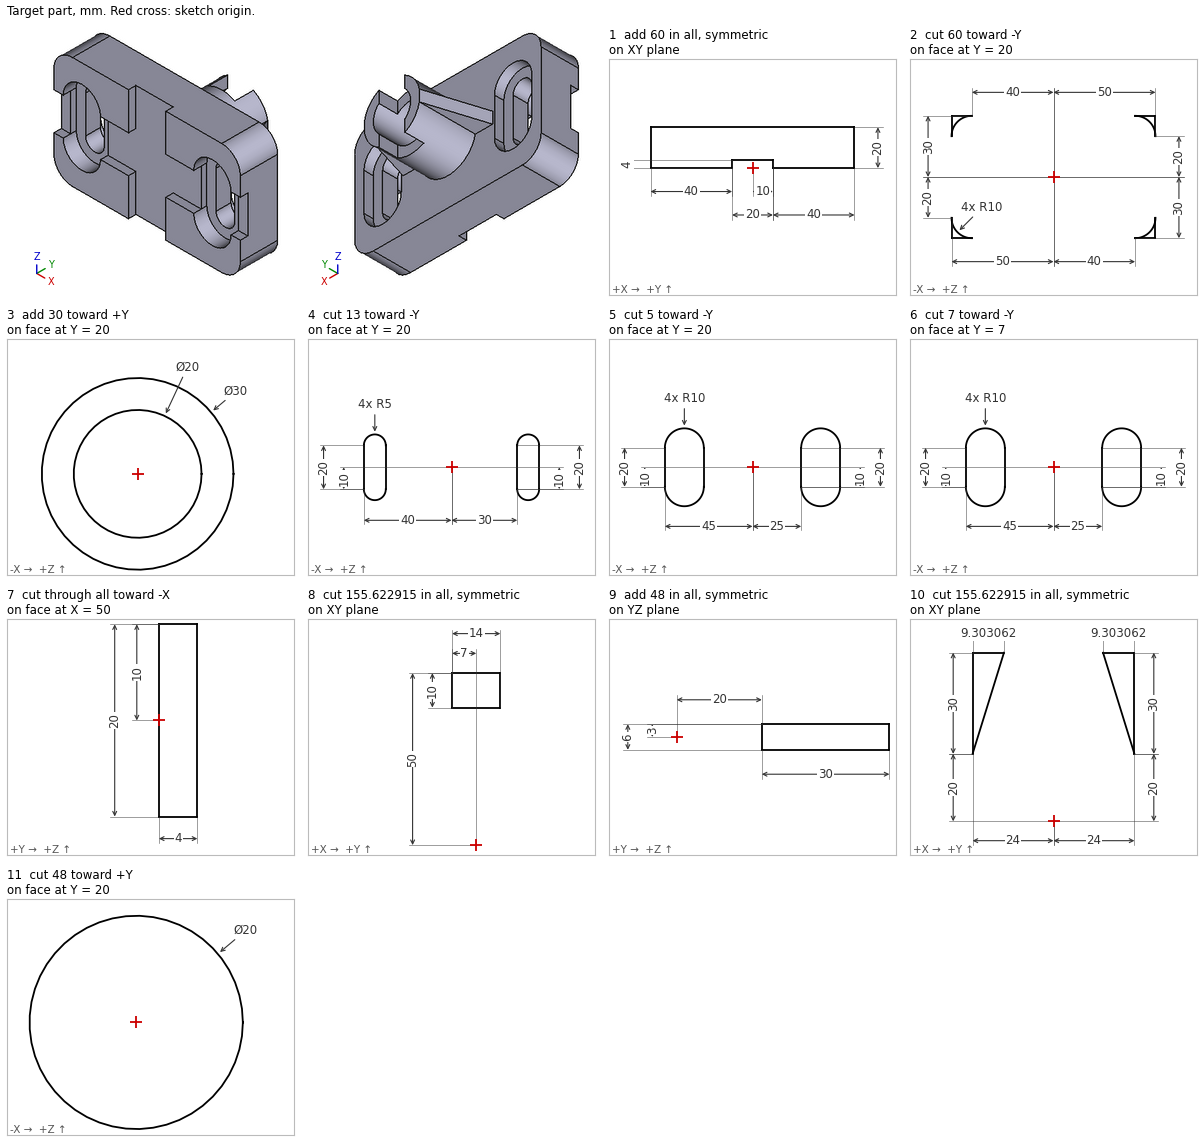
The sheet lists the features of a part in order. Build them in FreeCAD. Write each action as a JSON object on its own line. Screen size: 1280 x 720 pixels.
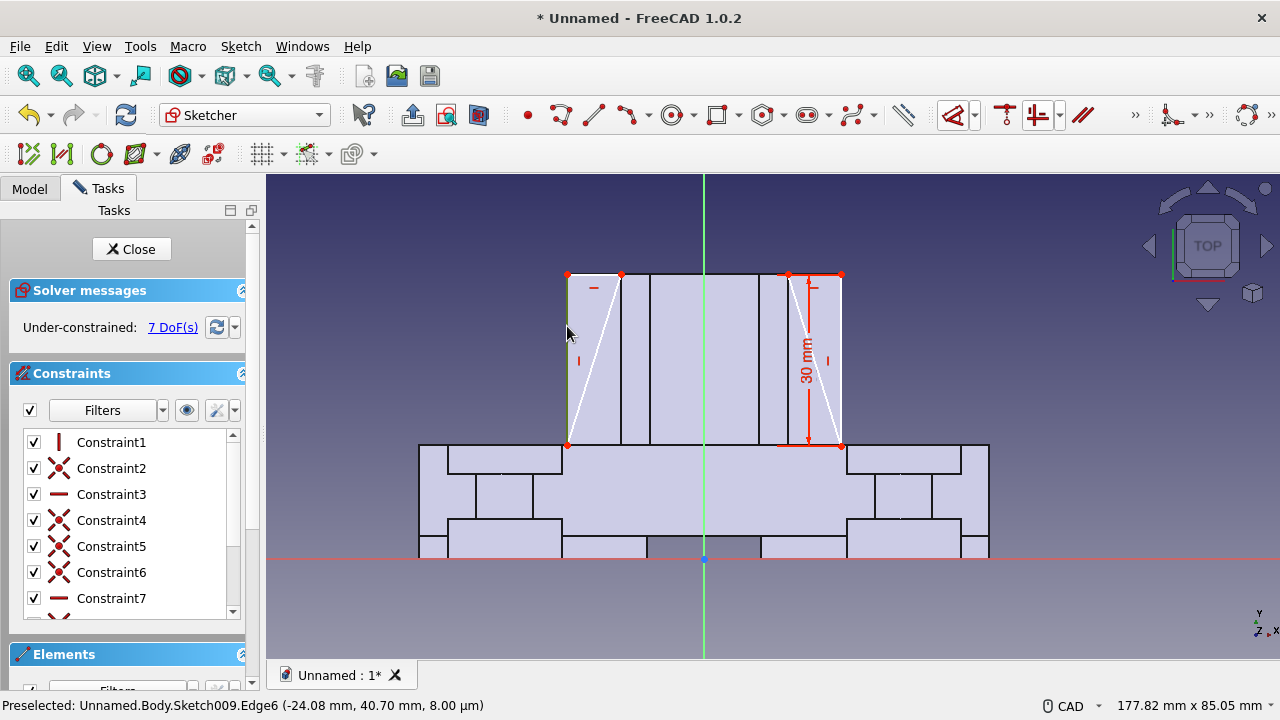
{"action": "left_click", "coordinate": [974, 116]}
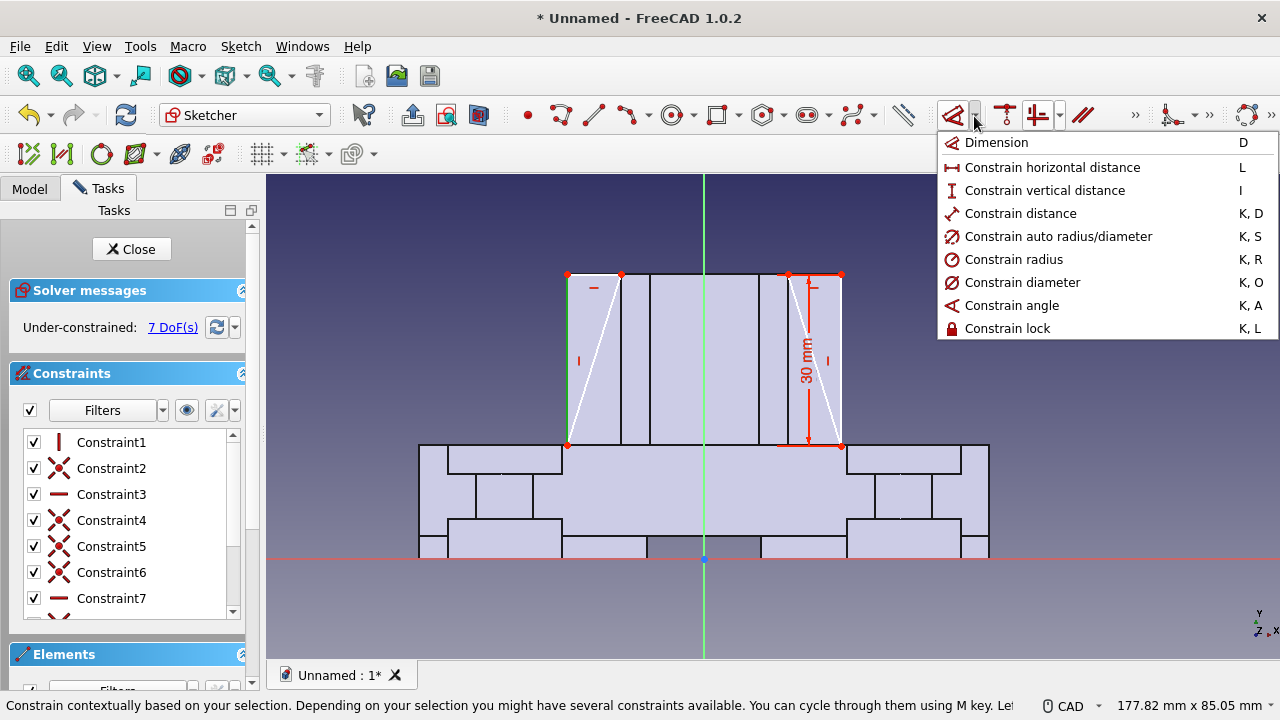
{"action": "left_click", "coordinate": [1108, 190]}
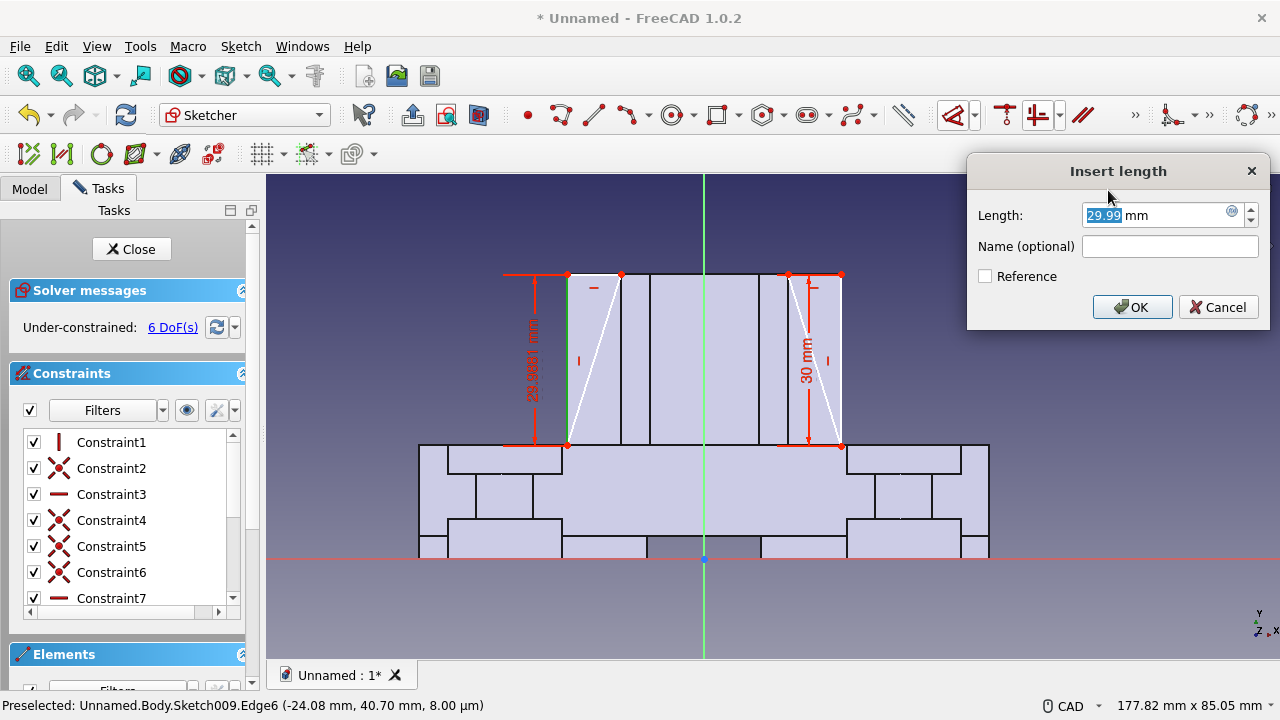
{"action": "type", "text": "30"}
{"action": "key", "text": "Return"}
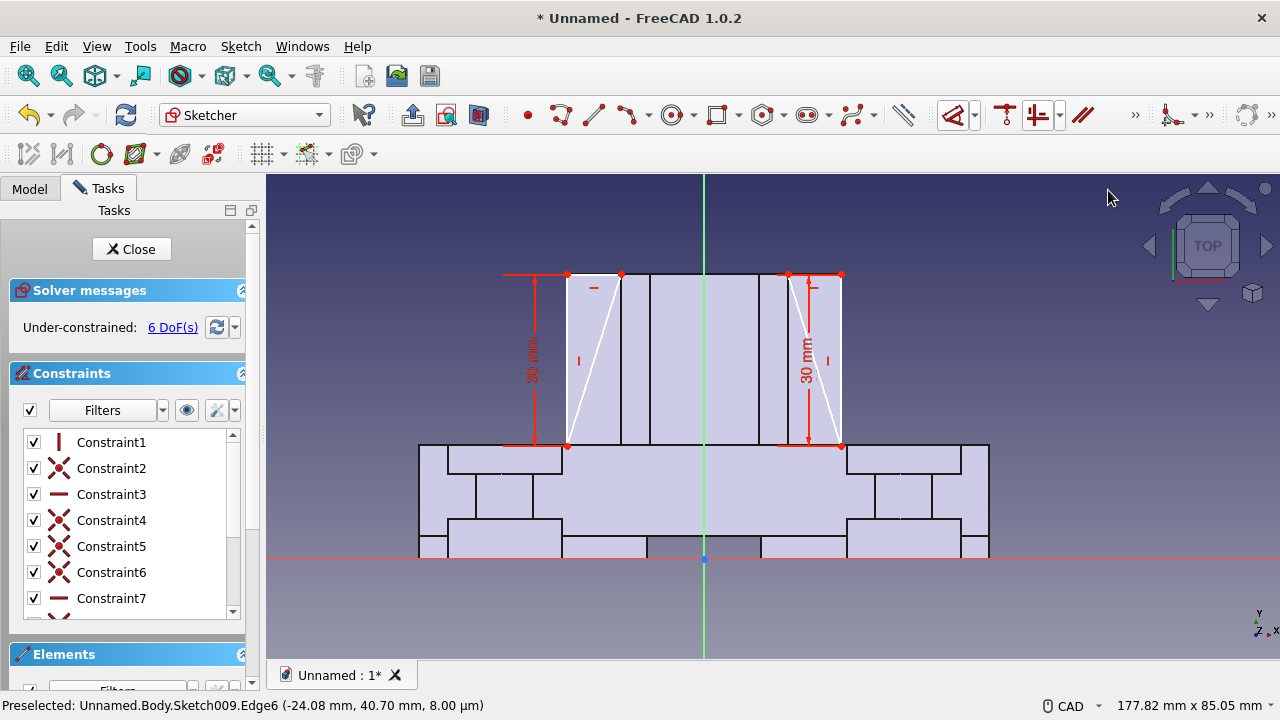
{"action": "left_click", "coordinate": [841, 446]}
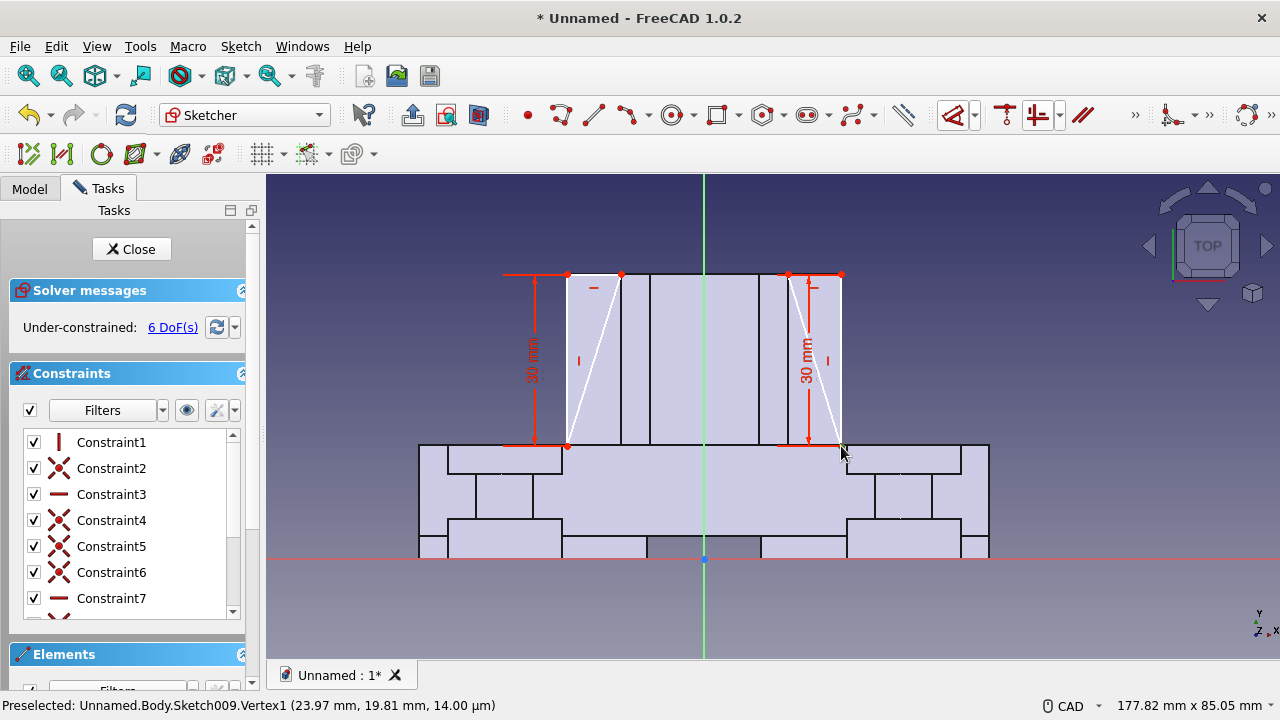
{"action": "key", "text": "l"}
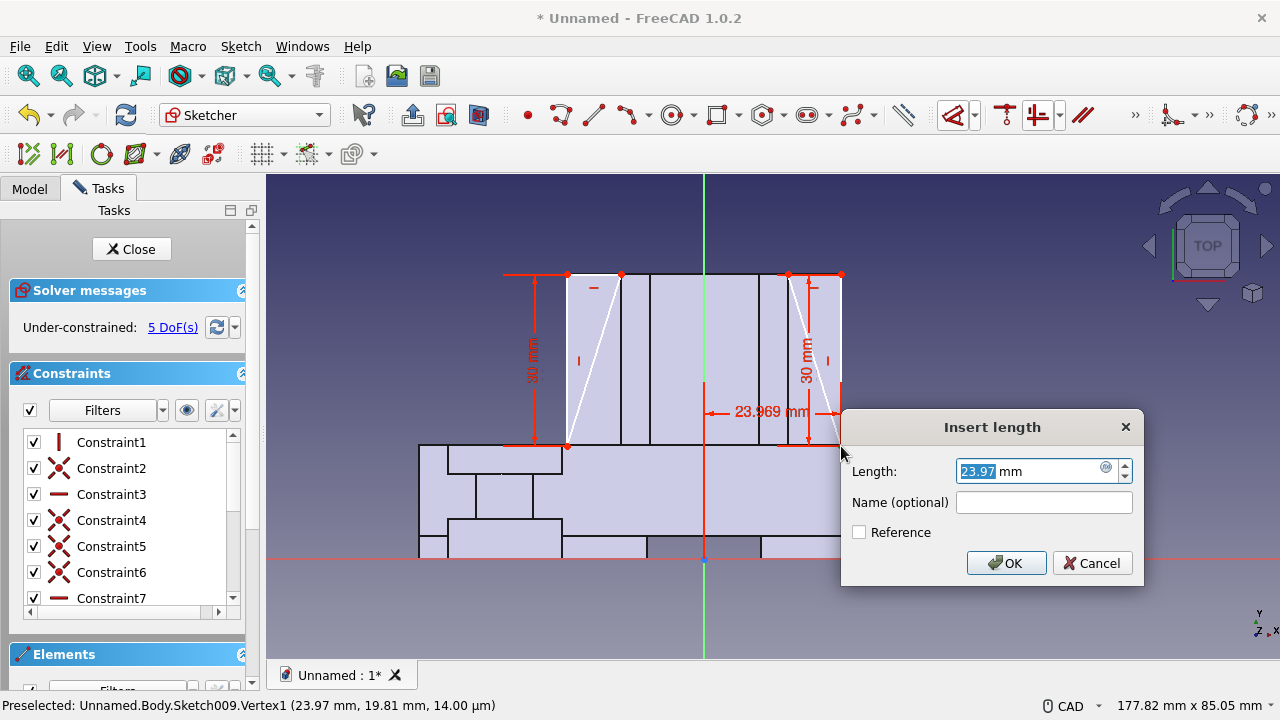
{"action": "type", "text": "24"}
{"action": "key", "text": "Return"}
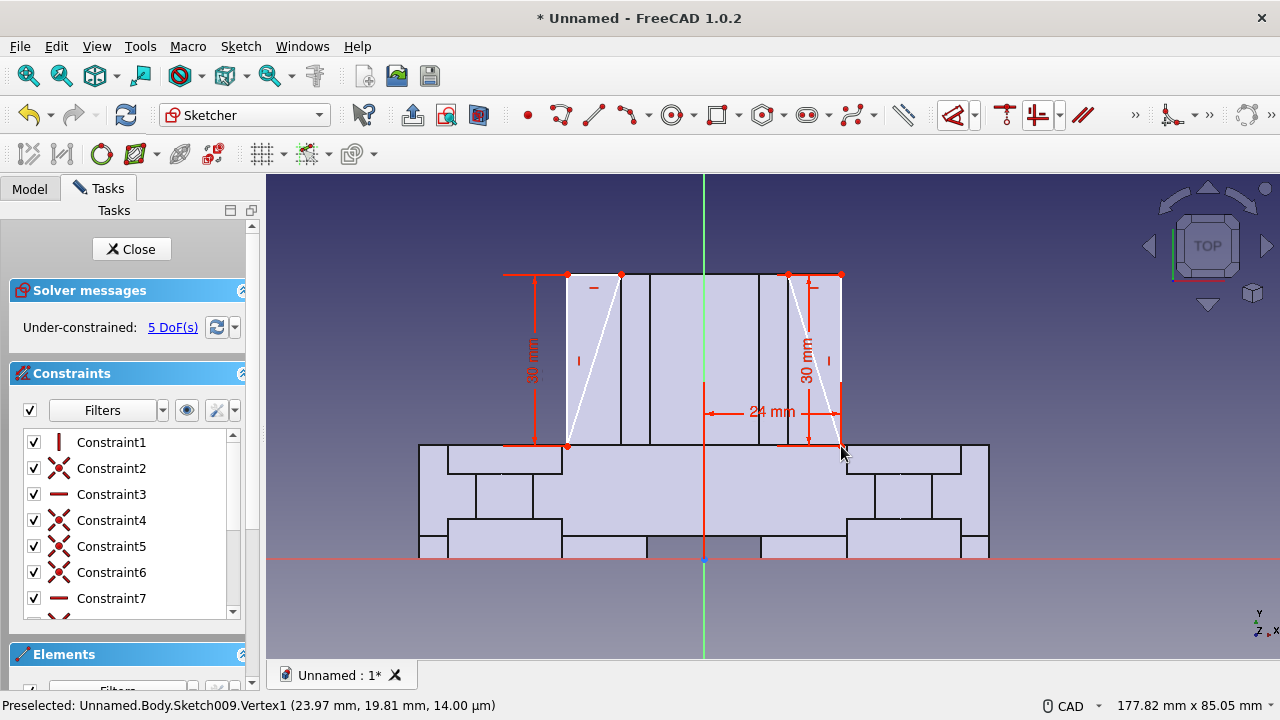
{"action": "left_click", "coordinate": [841, 446]}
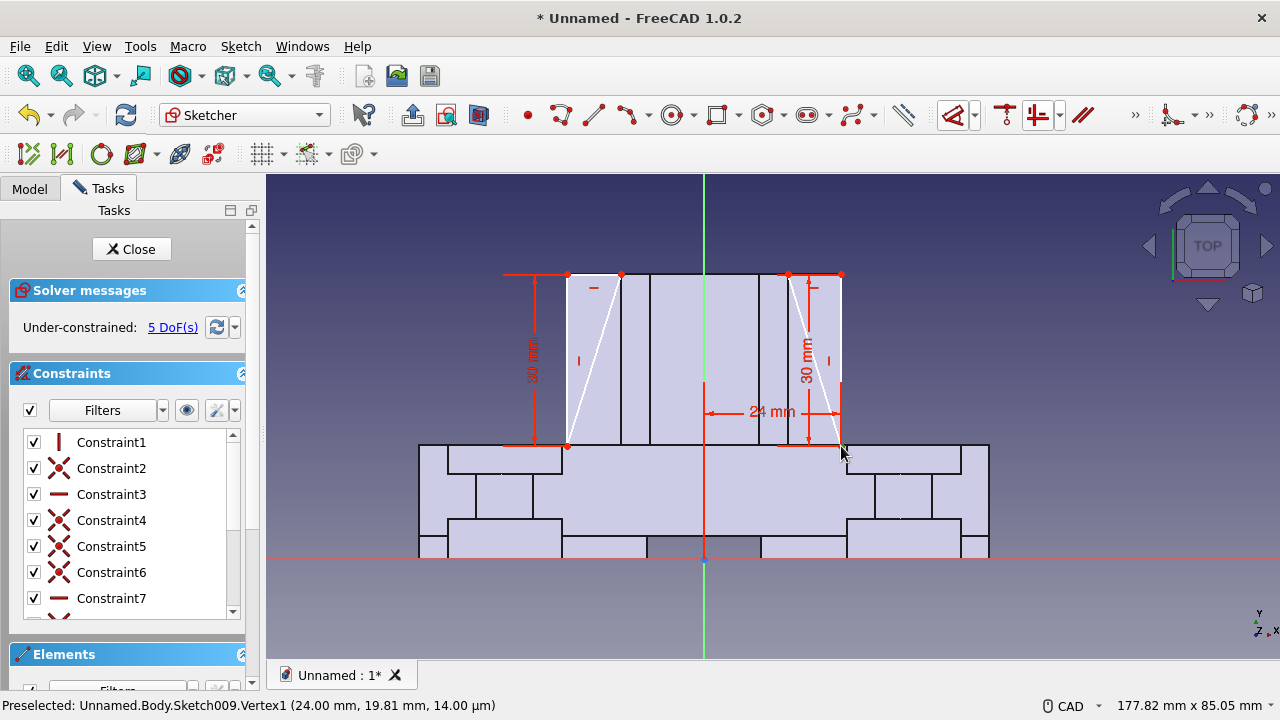
{"action": "key", "text": "i"}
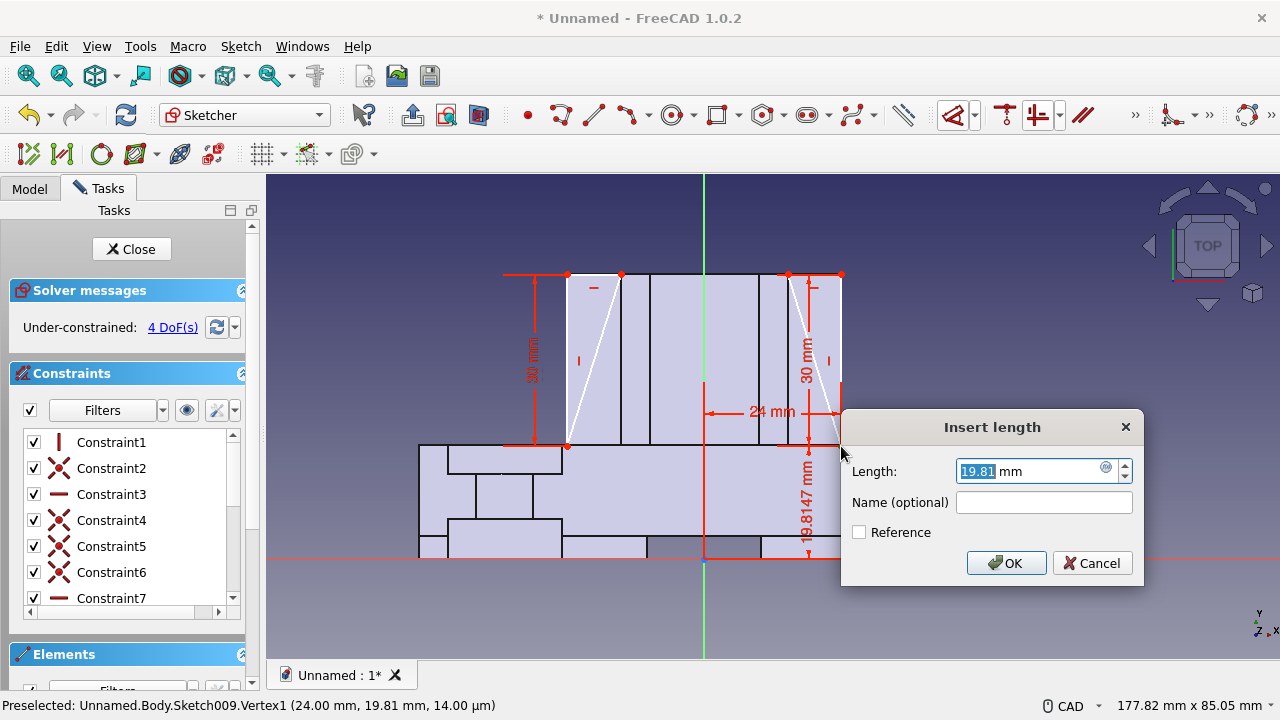
{"action": "type", "text": "20"}
{"action": "key", "text": "Return"}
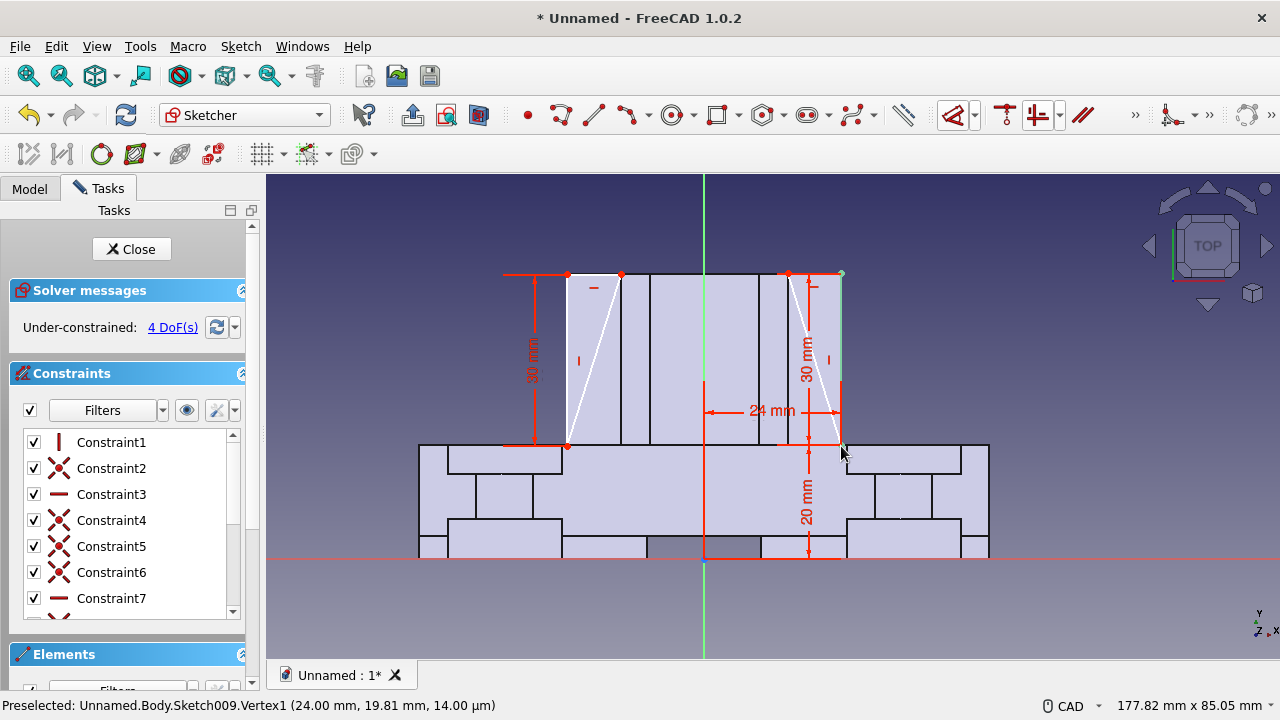
{"action": "left_click", "coordinate": [567, 446]}